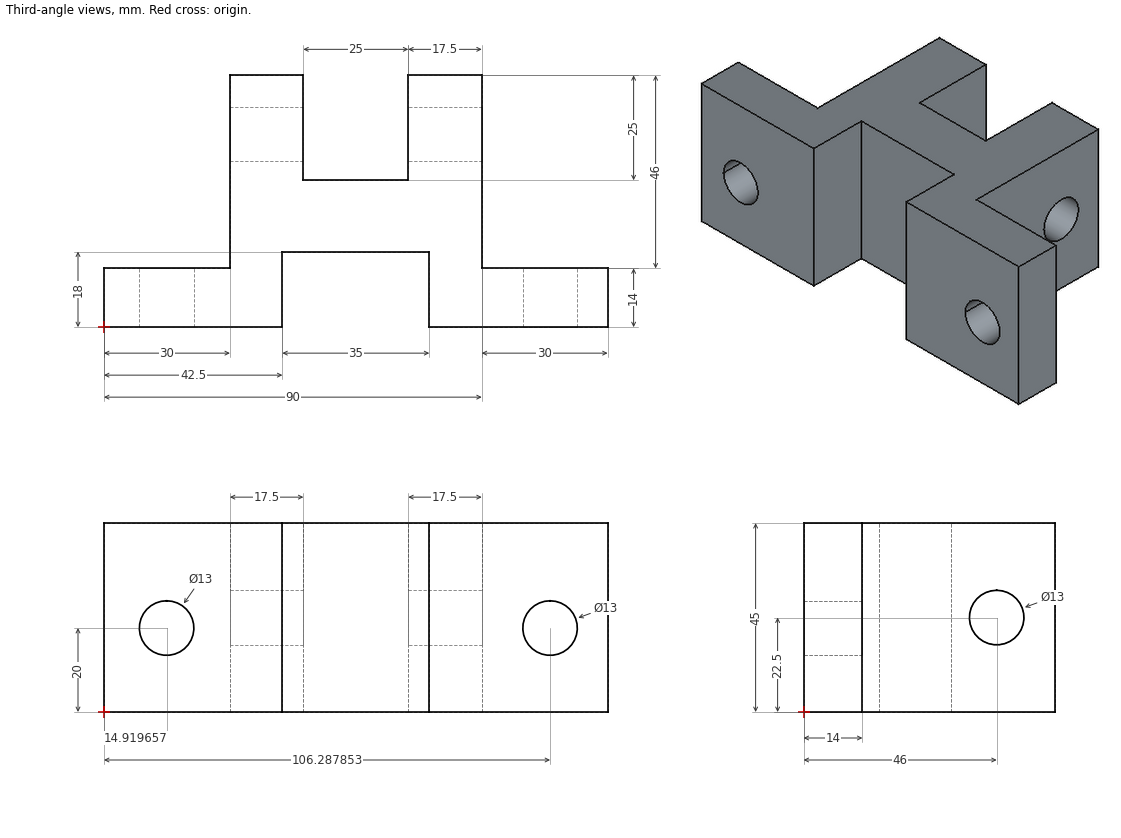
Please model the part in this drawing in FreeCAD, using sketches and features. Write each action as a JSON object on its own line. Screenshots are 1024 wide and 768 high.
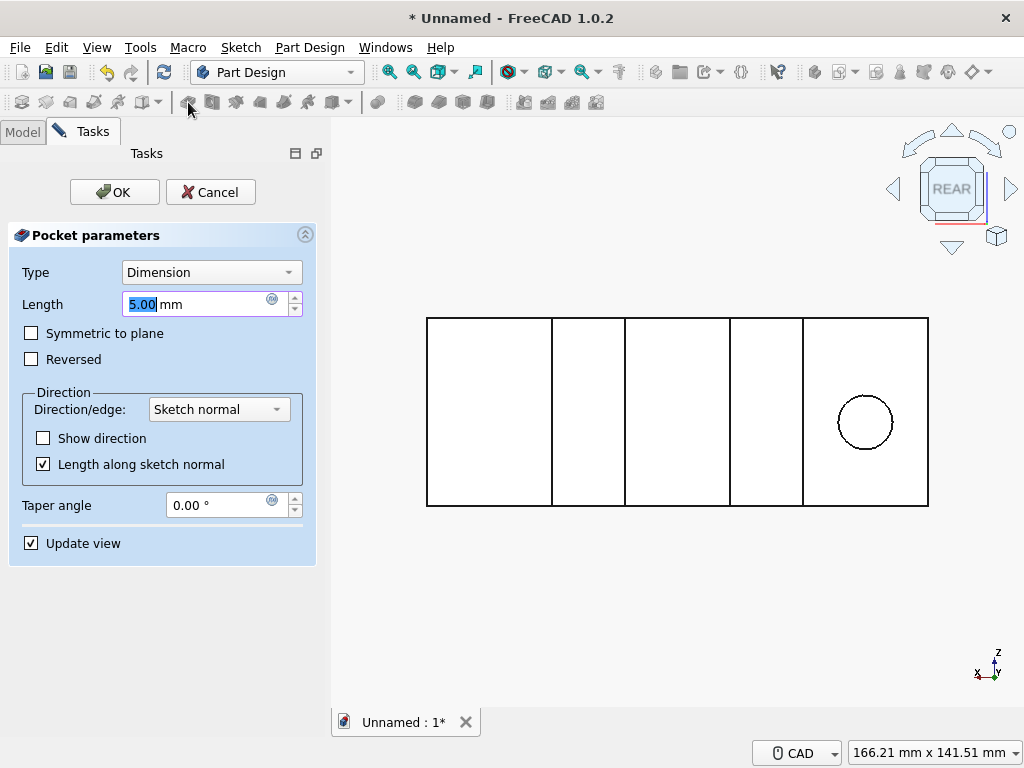
{"action": "type", "text": "14"}
{"action": "key", "text": "Tab"}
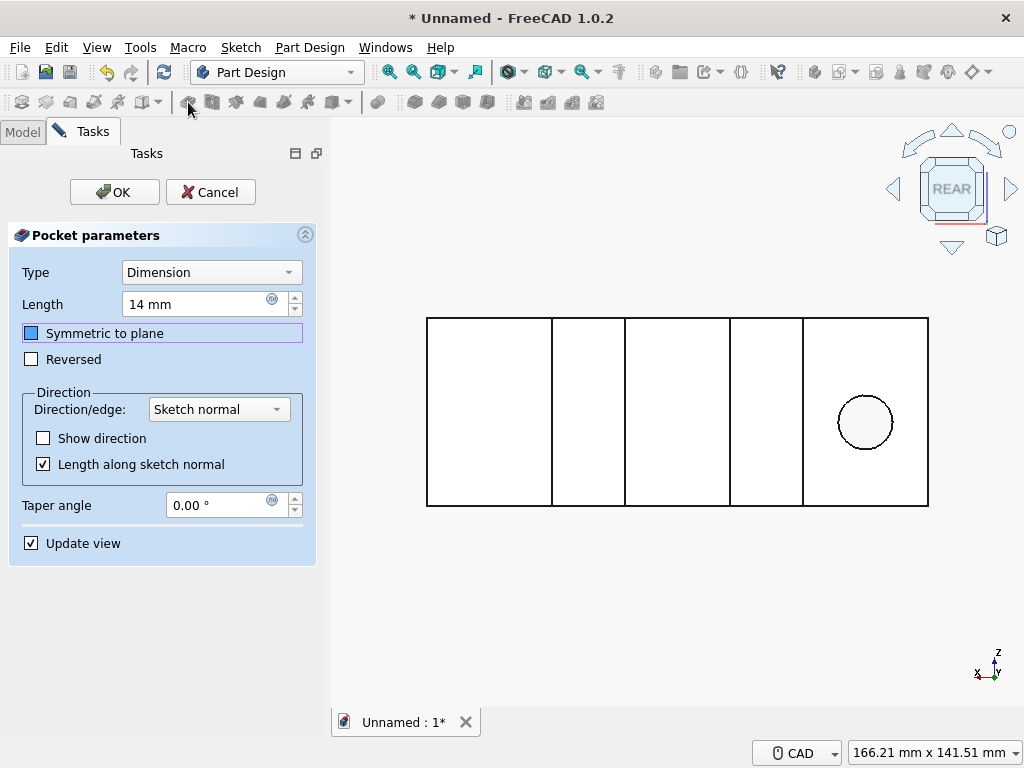
{"action": "left_click", "coordinate": [115, 192]}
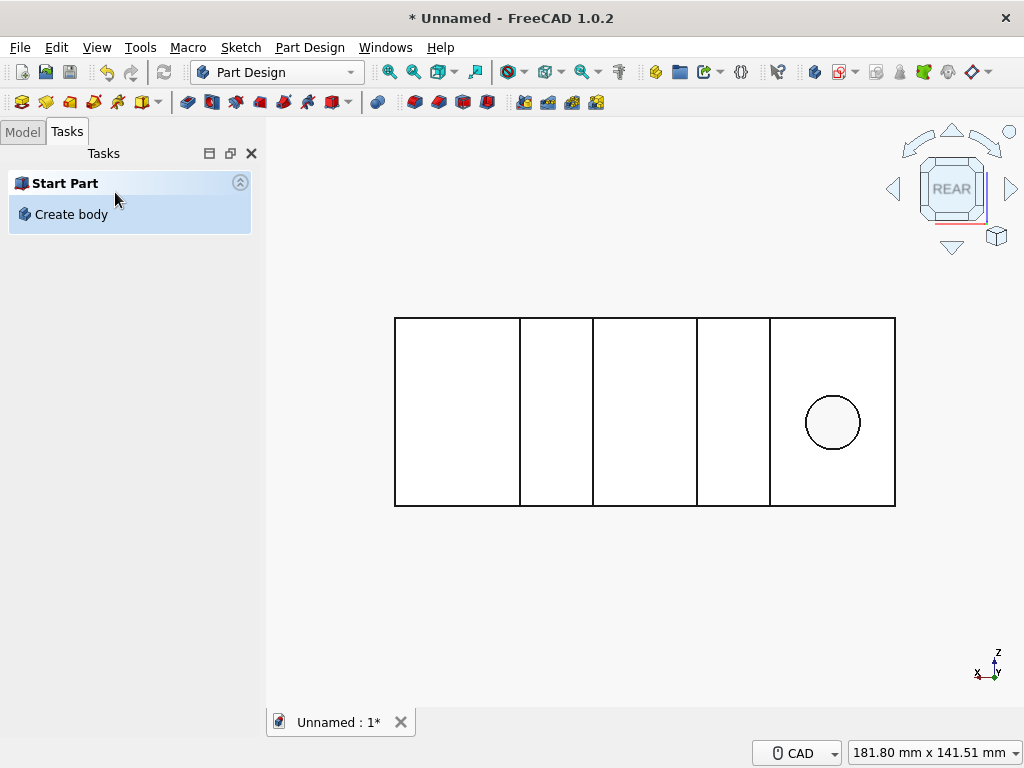
{"action": "left_click", "coordinate": [457, 384]}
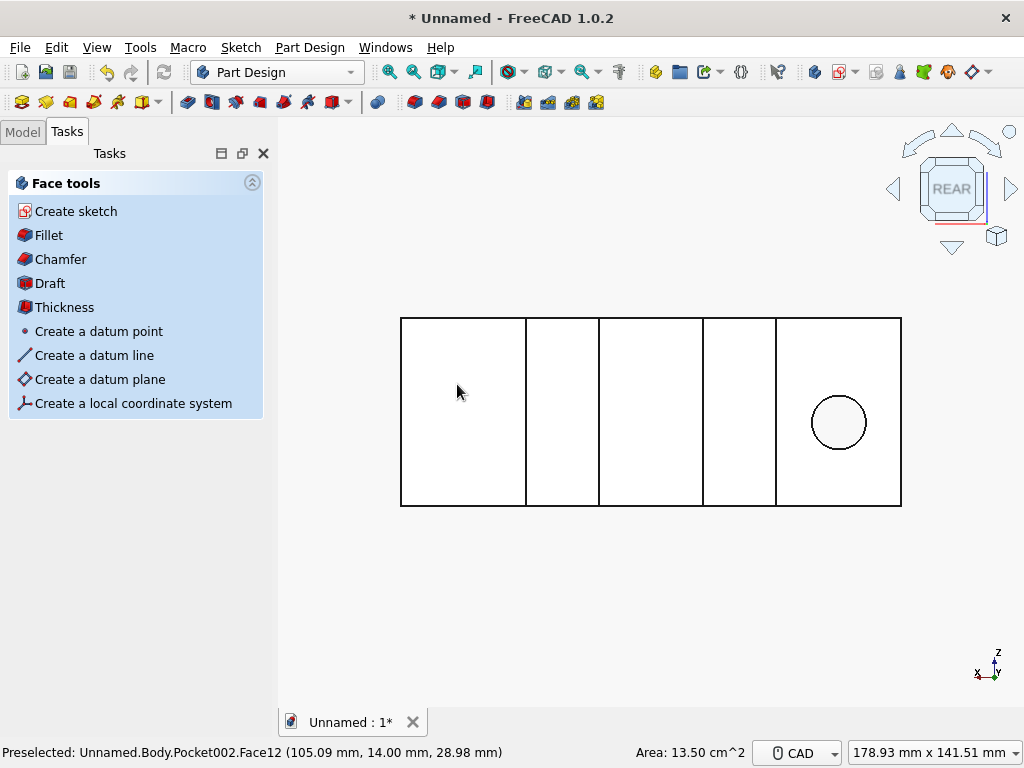
{"action": "left_click", "coordinate": [840, 72]}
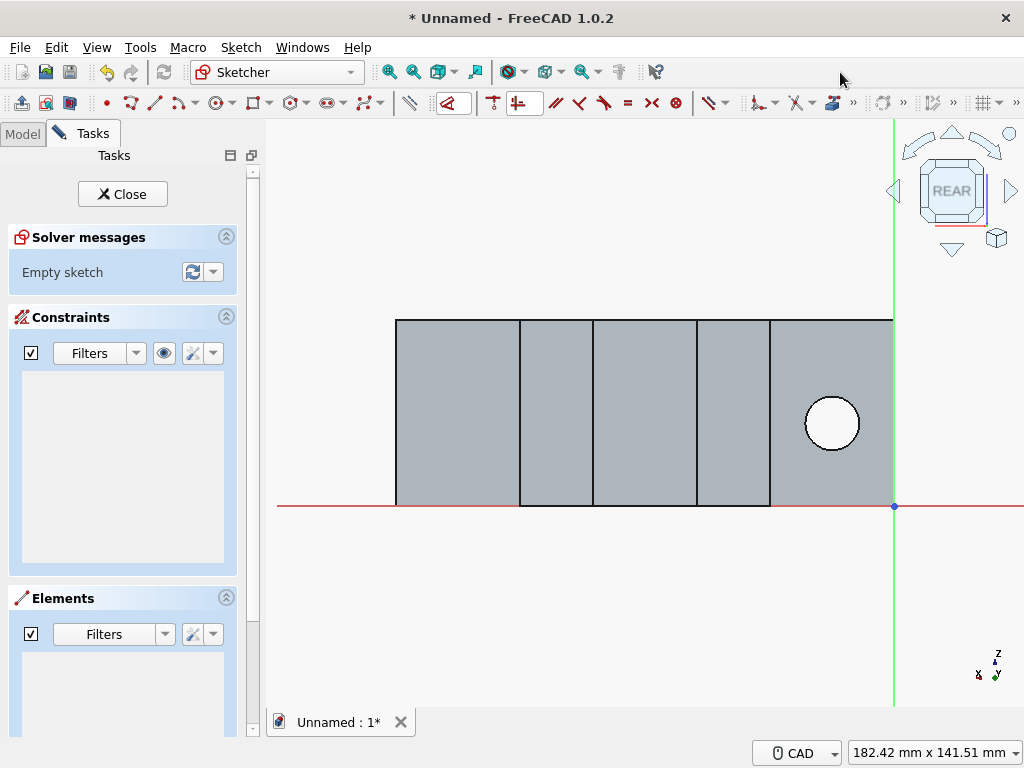
{"action": "left_click", "coordinate": [70, 104]}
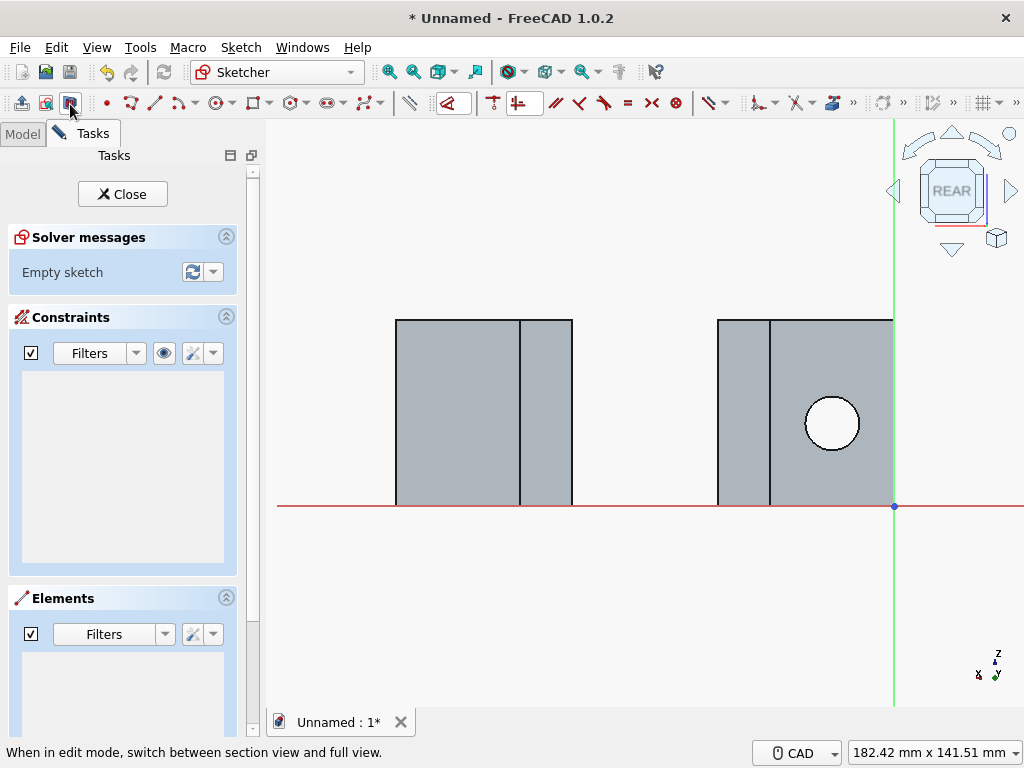
{"action": "scroll", "coordinate": [433, 425], "scroll_direction": "up", "scroll_amount": 10}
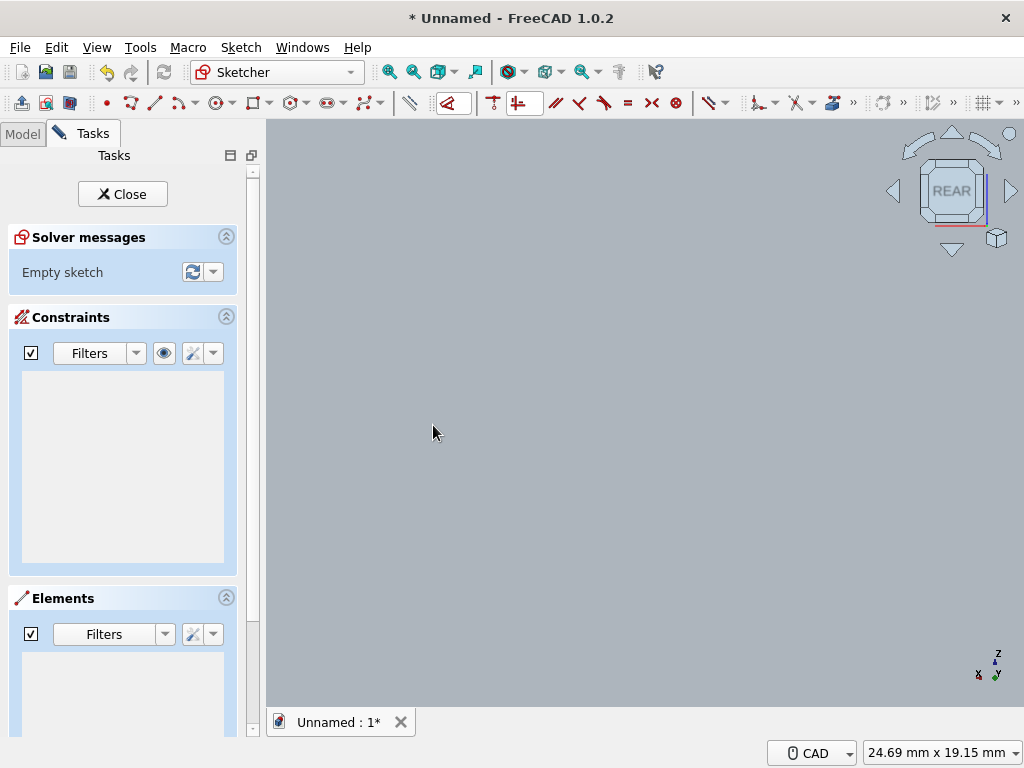
{"action": "key", "text": "g c"}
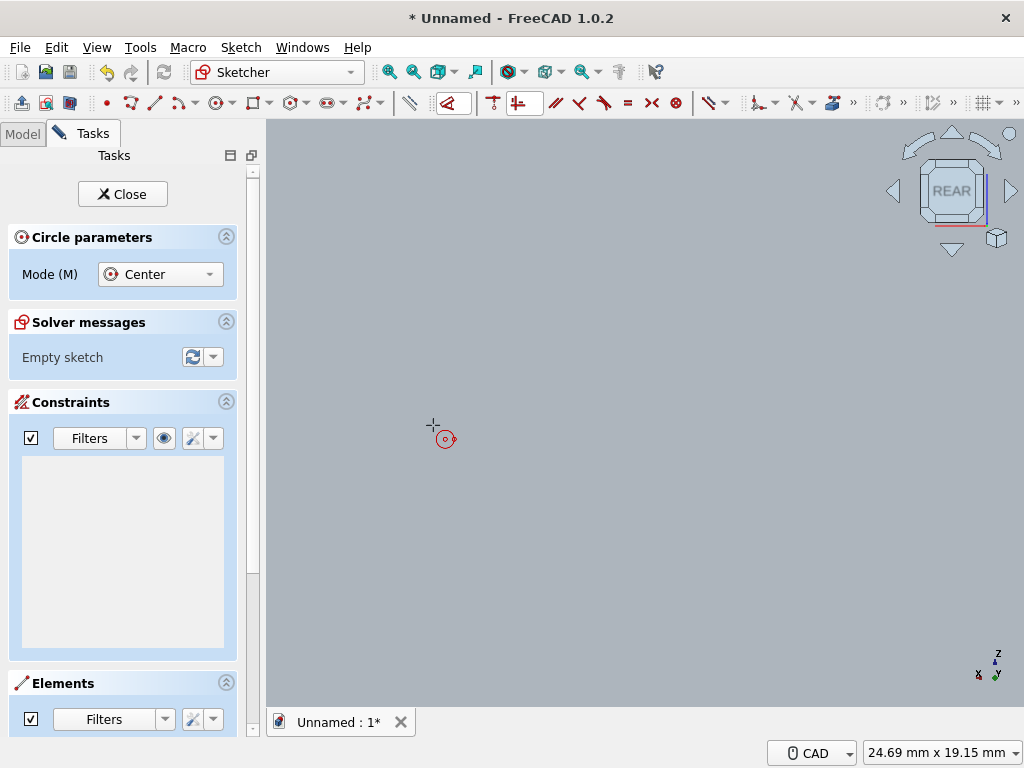
{"action": "left_click", "coordinate": [577, 410]}
{"action": "mouse_move", "coordinate": [718, 269]}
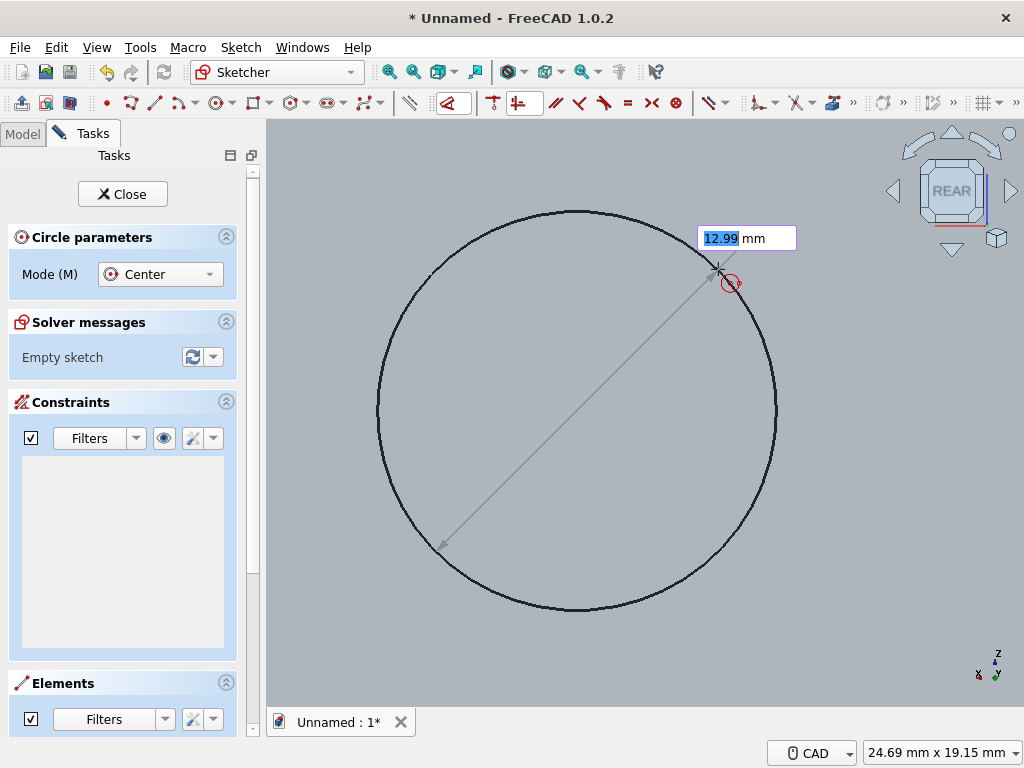
{"action": "type", "text": "13"}
{"action": "key", "text": "Return"}
{"action": "key", "text": "Escape"}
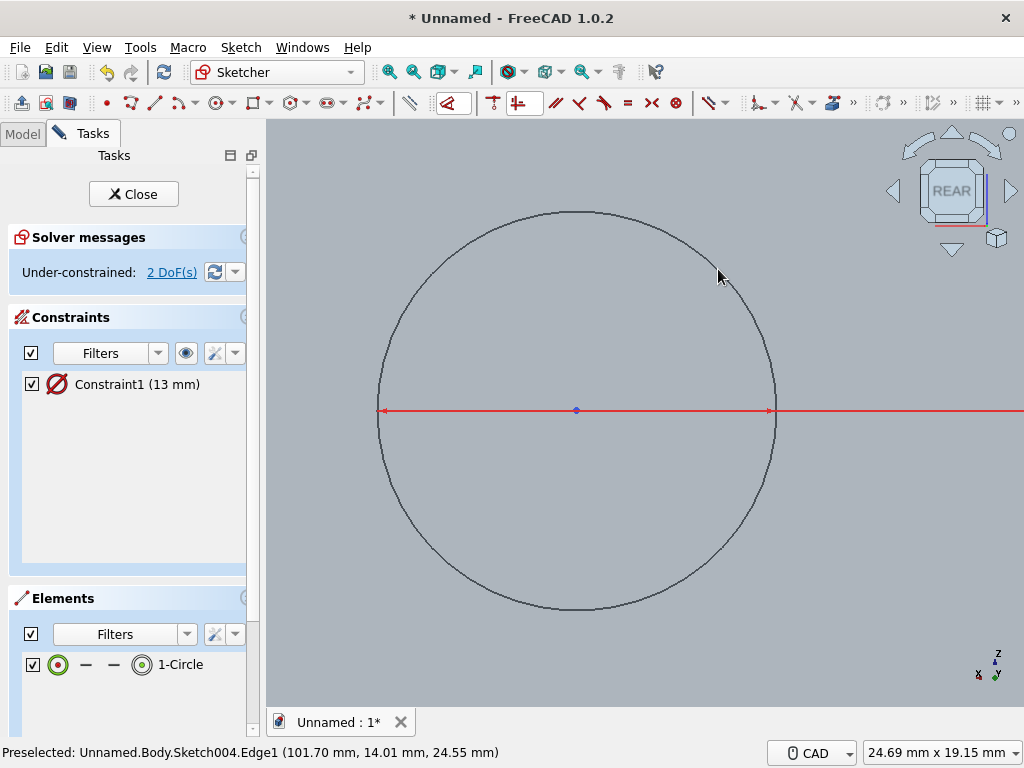
{"action": "left_click", "coordinate": [577, 411]}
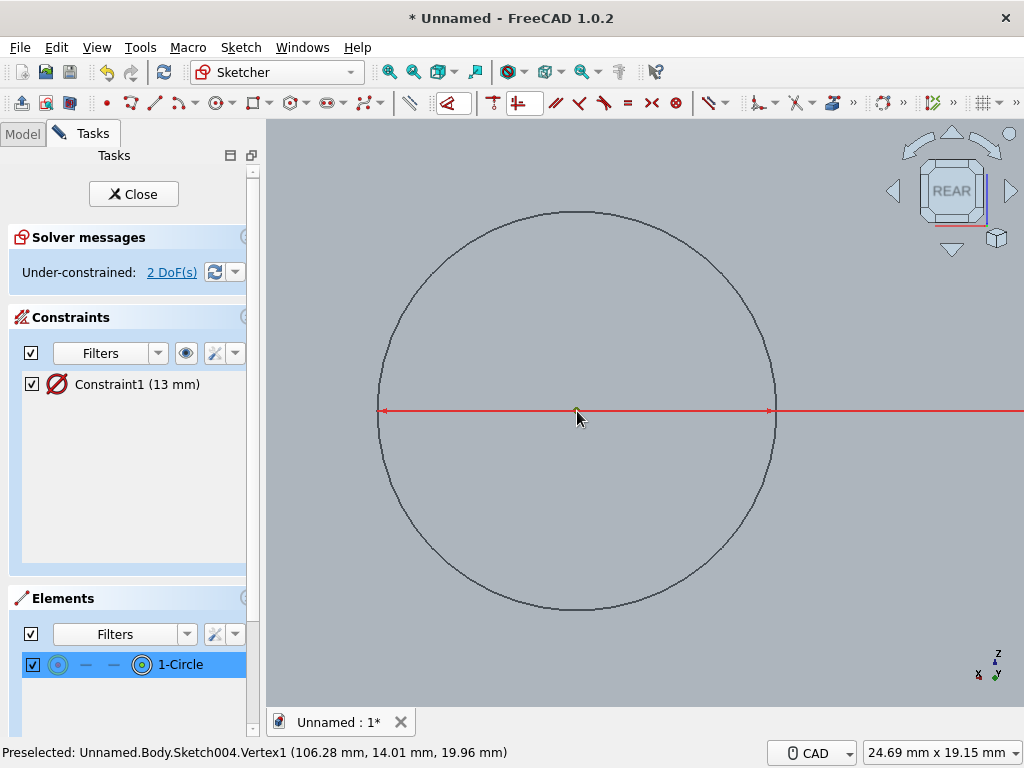
{"action": "key", "text": "i"}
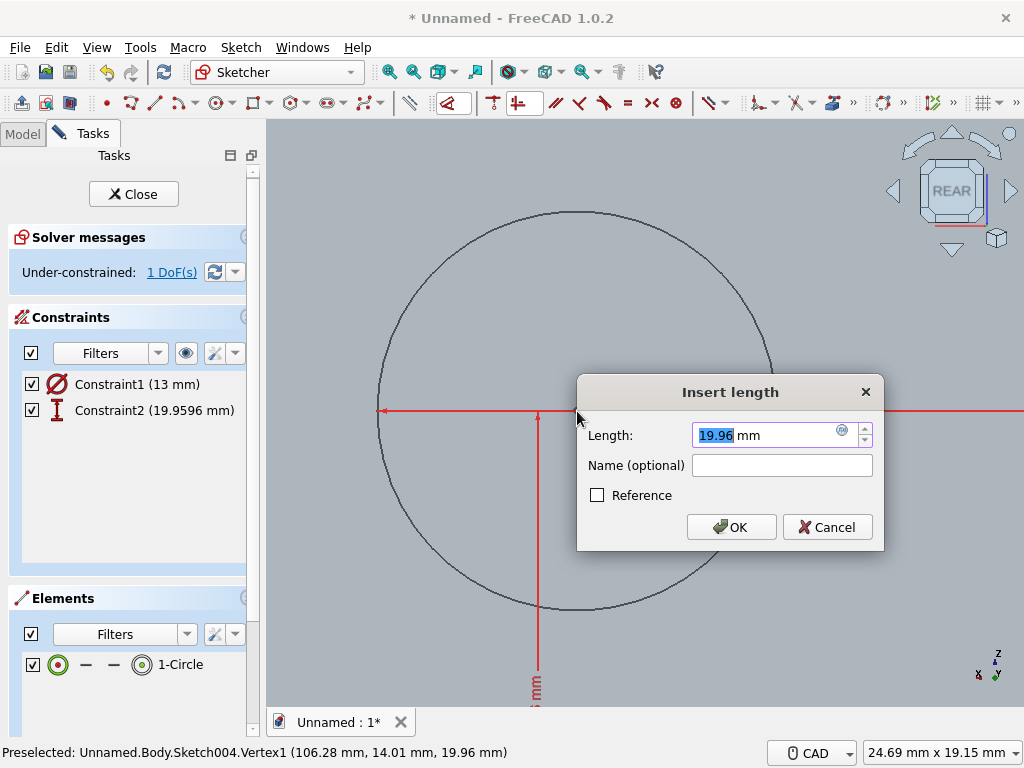
{"action": "type", "text": "20"}
{"action": "key", "text": "Return"}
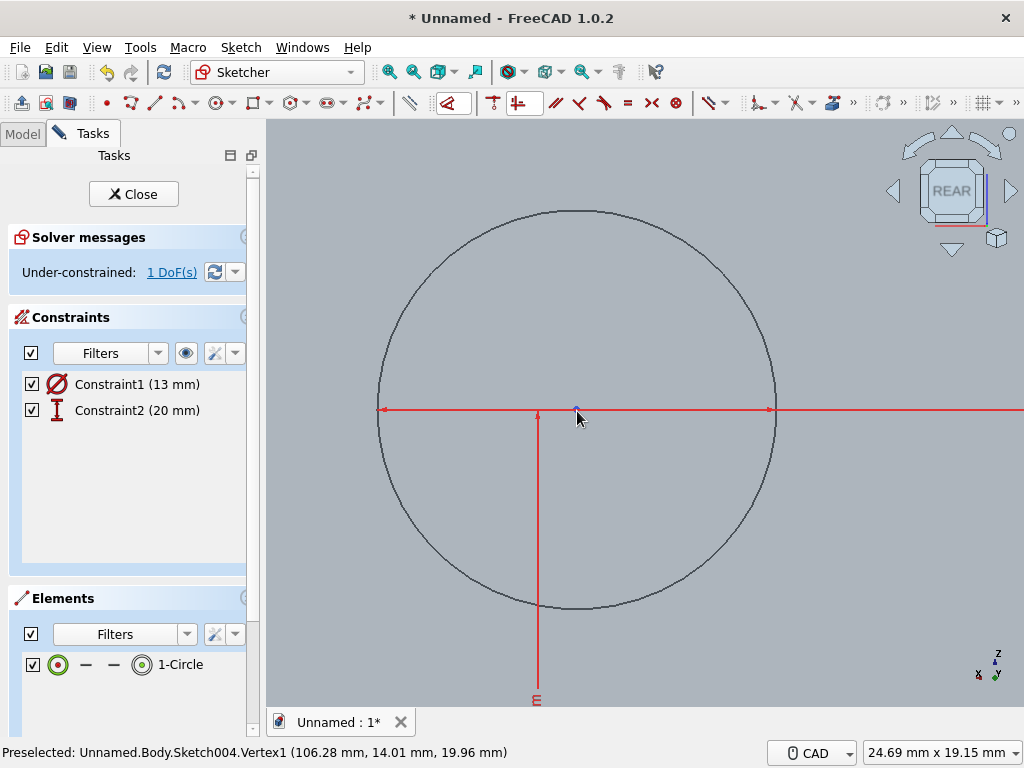
{"action": "left_click", "coordinate": [577, 410]}